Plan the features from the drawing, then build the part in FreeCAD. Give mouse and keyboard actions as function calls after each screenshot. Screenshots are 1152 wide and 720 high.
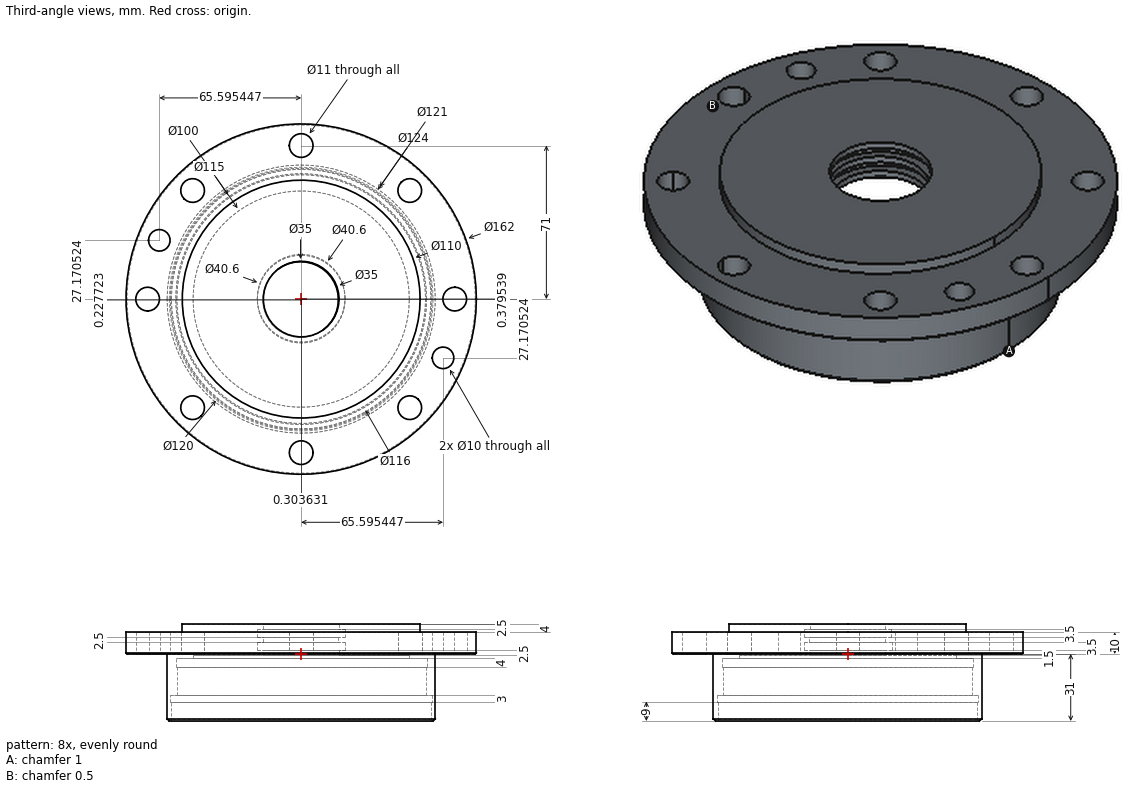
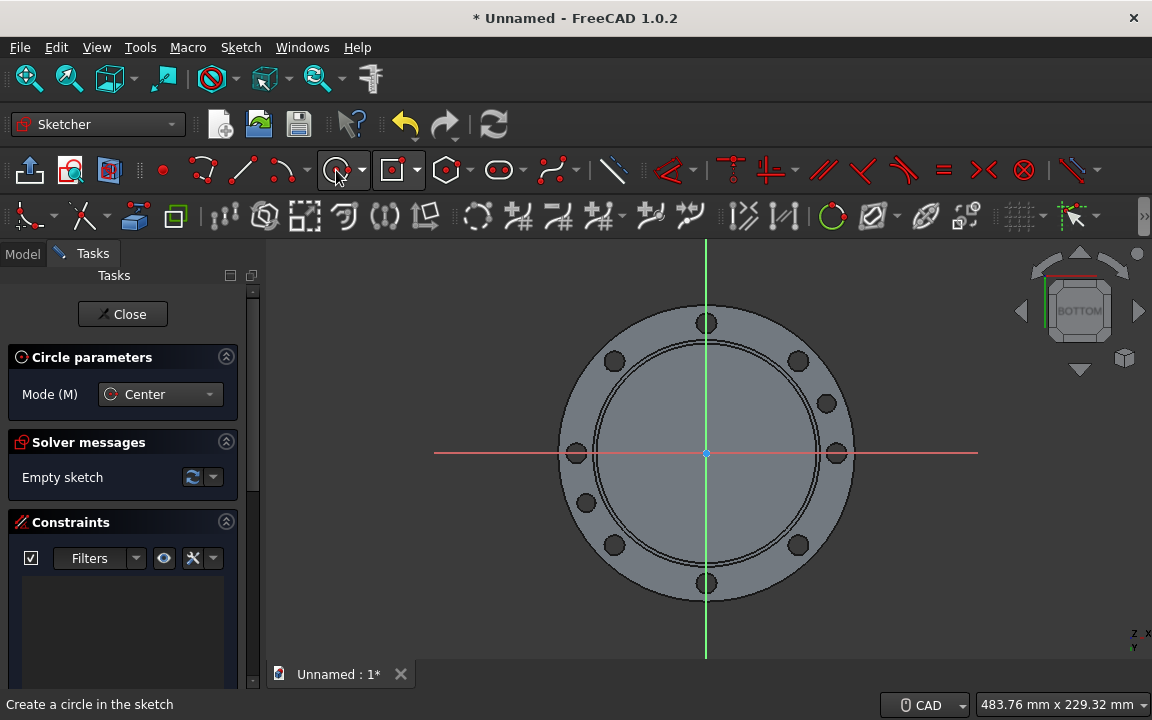
click(706, 453)
click(785, 375)
key(Escape)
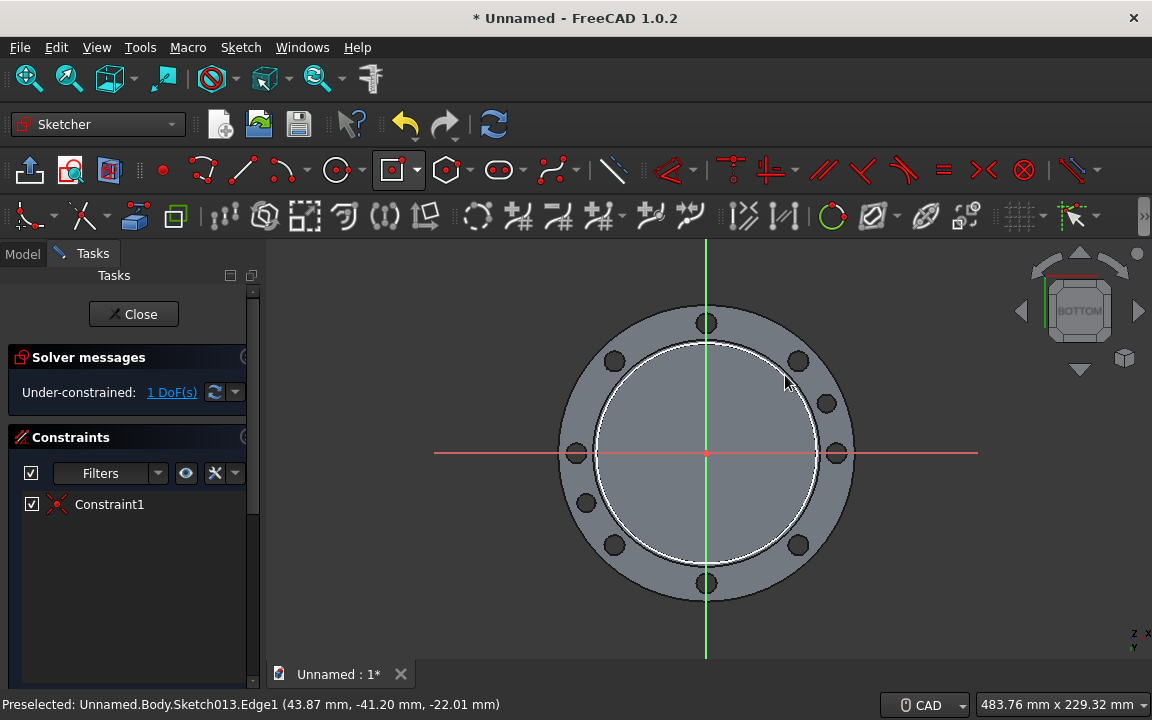
click(668, 170)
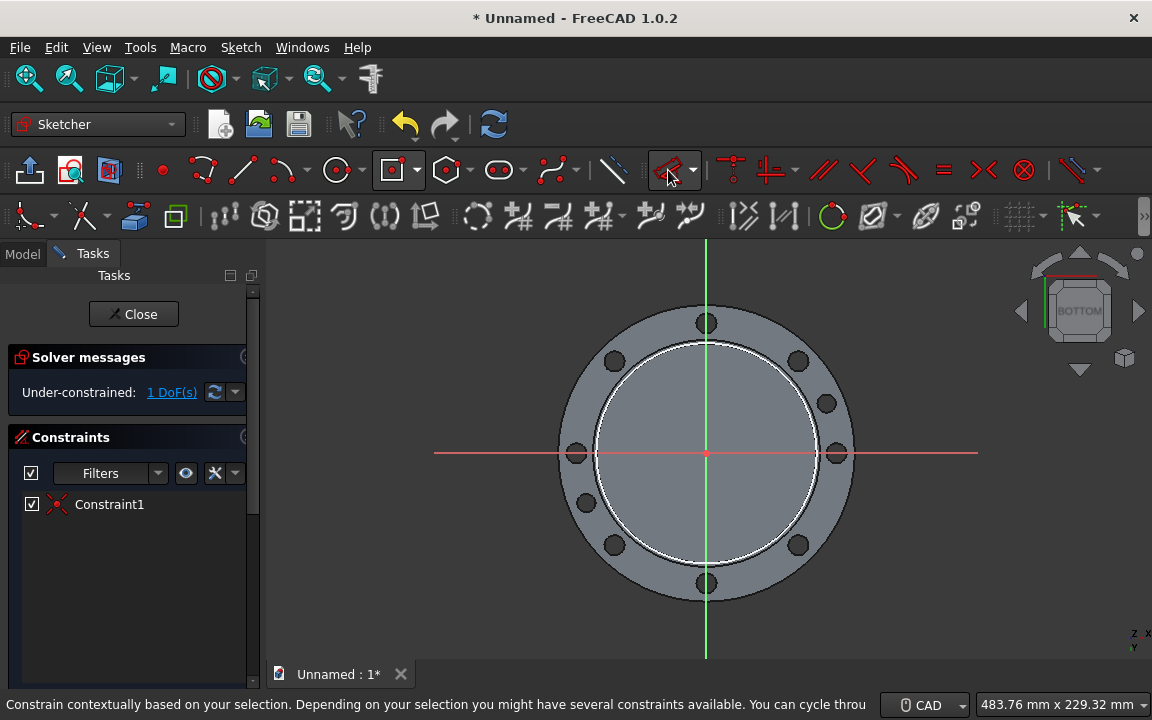
click(784, 375)
click(807, 352)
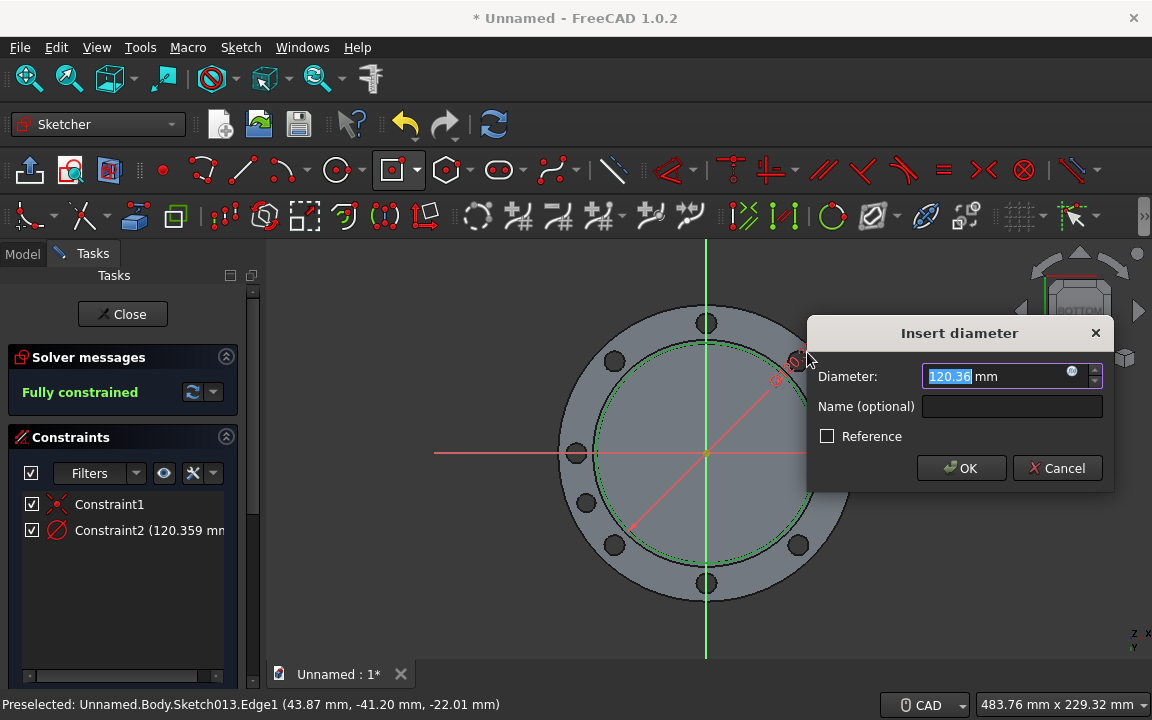
text(121)
key(Return)
key(Escape)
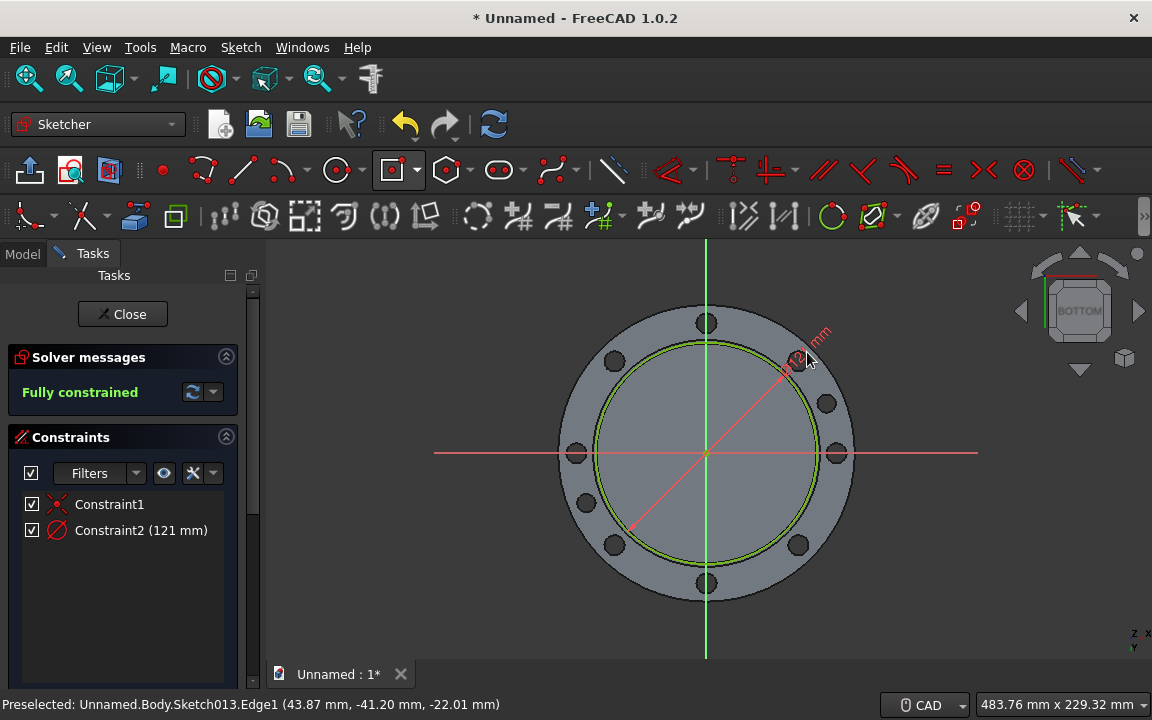
click(123, 314)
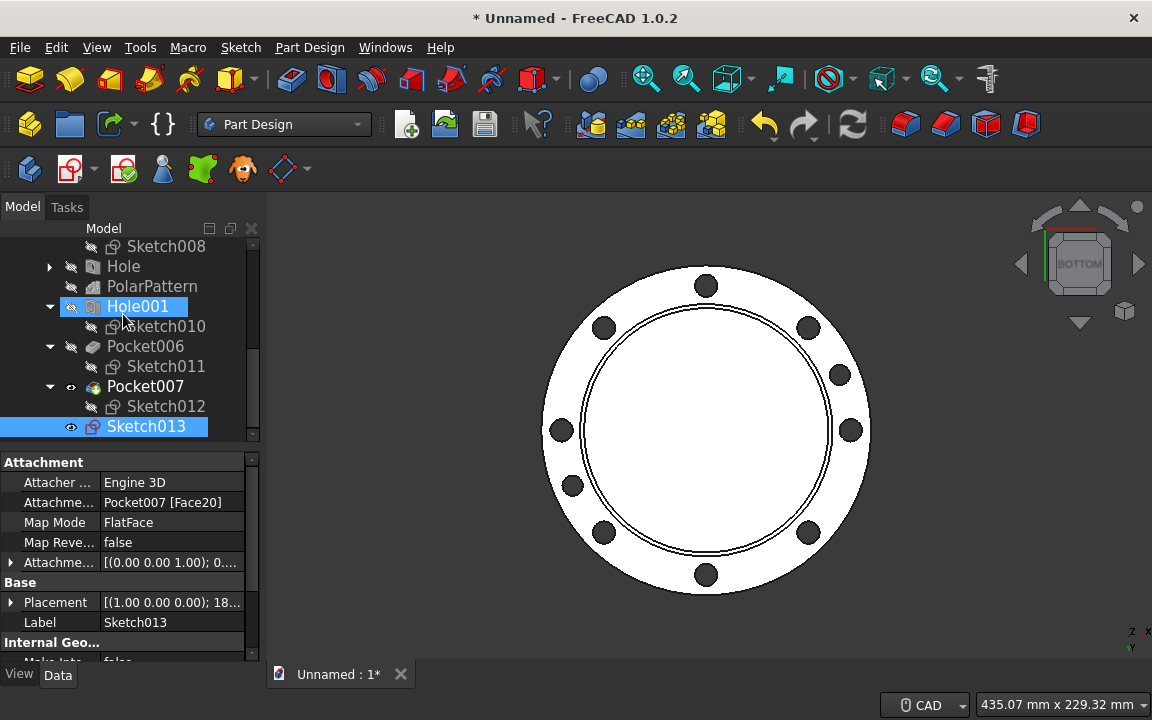
click(292, 80)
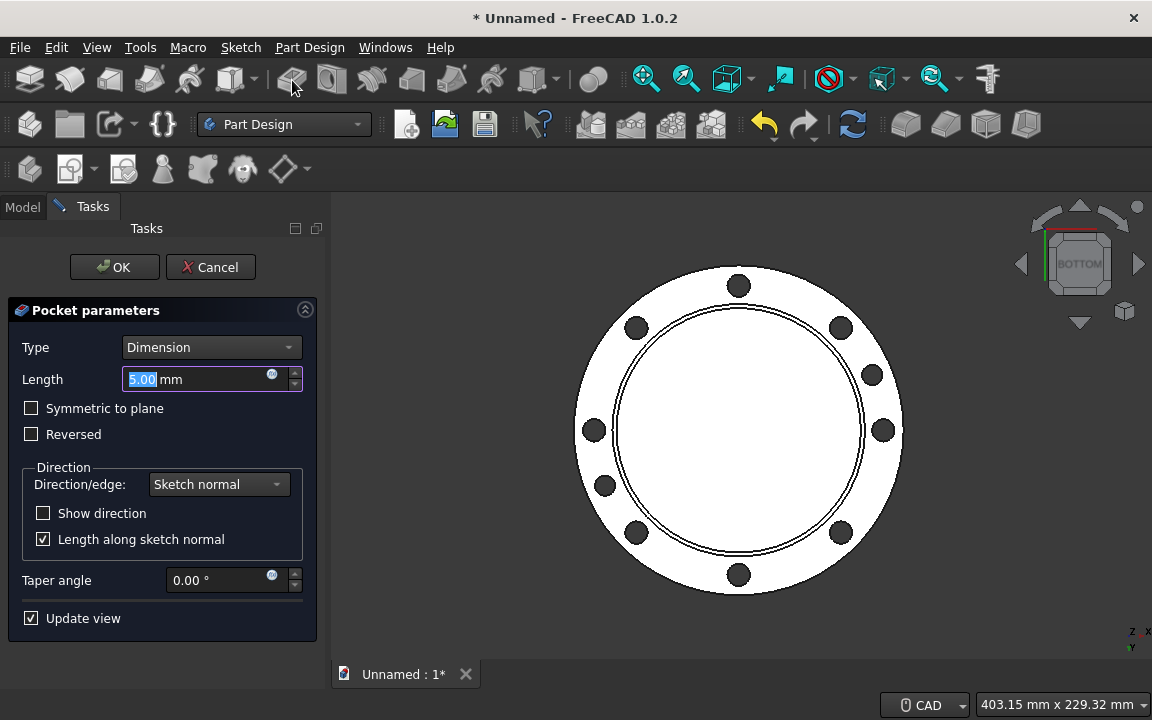
text(3)
key(Tab)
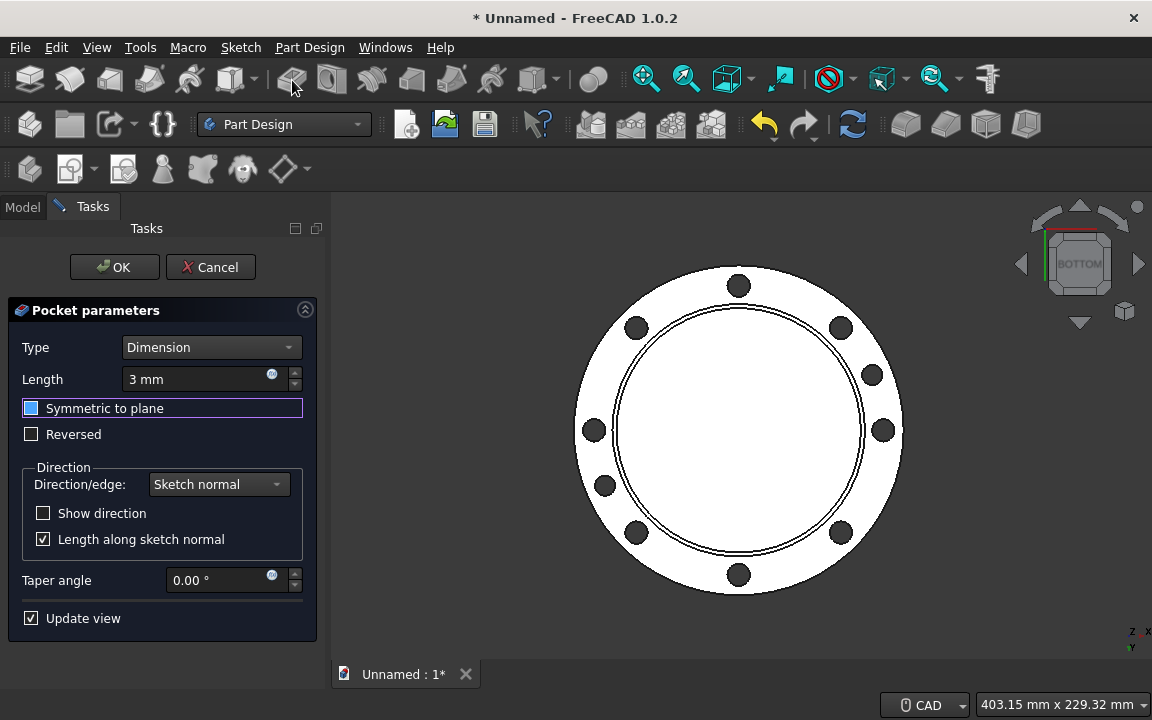
click(115, 267)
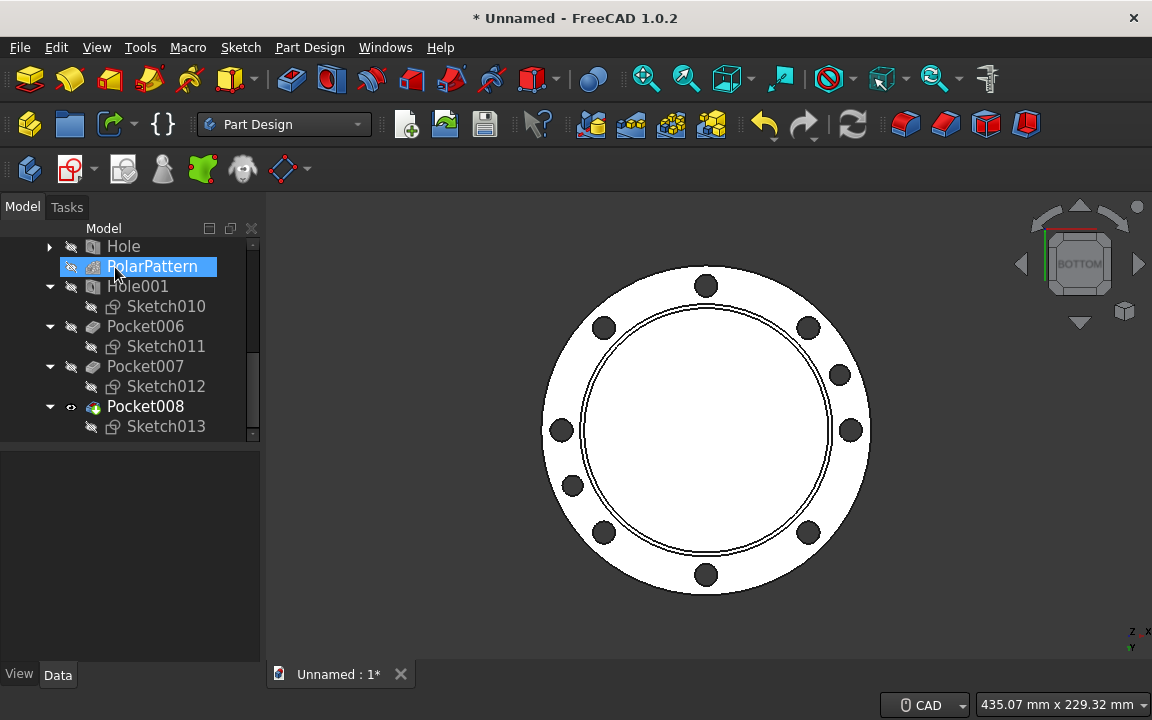
click(706, 429)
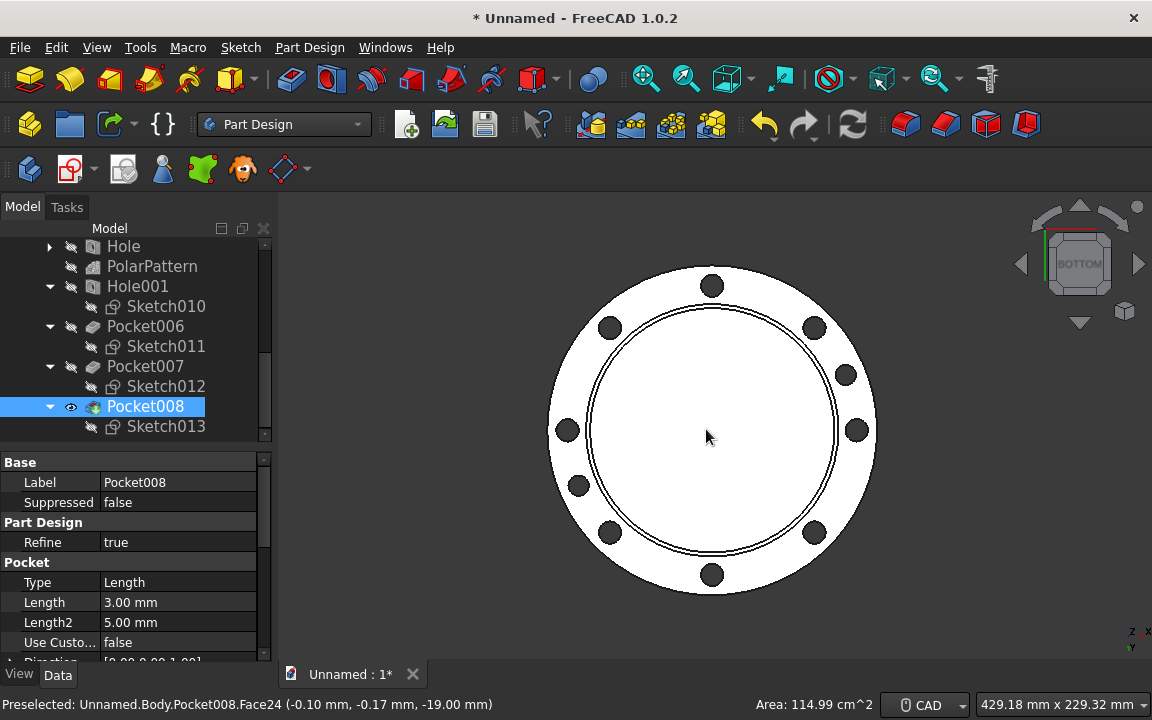
click(70, 170)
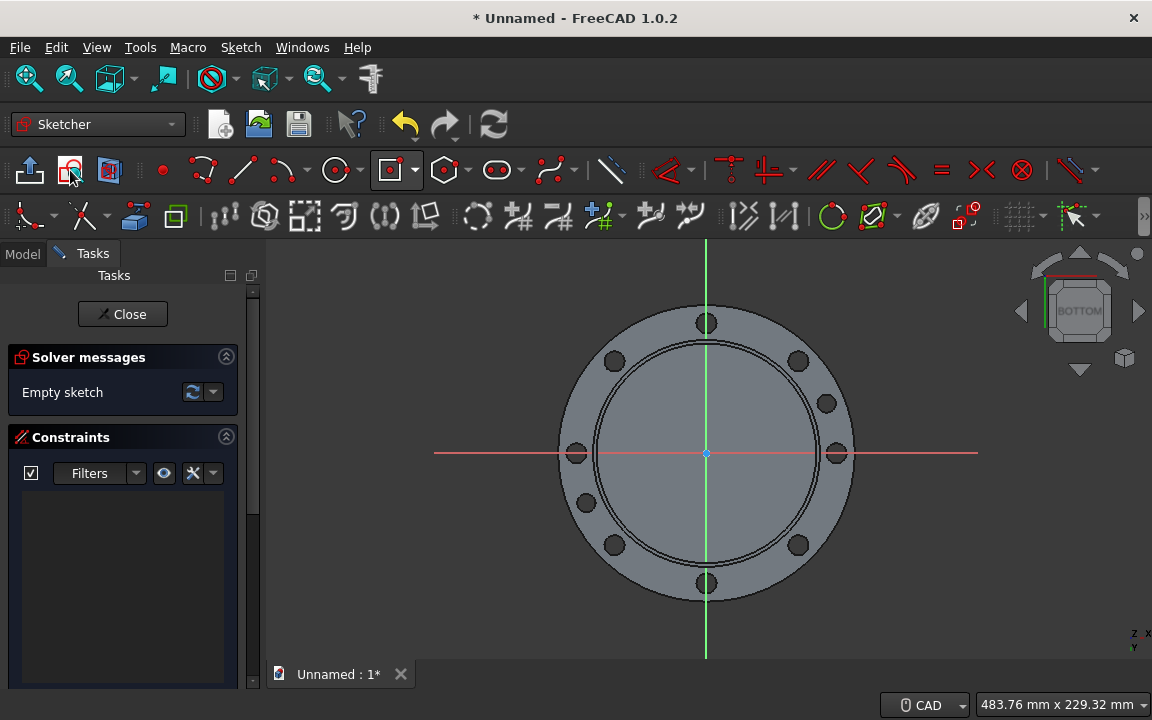
click(336, 170)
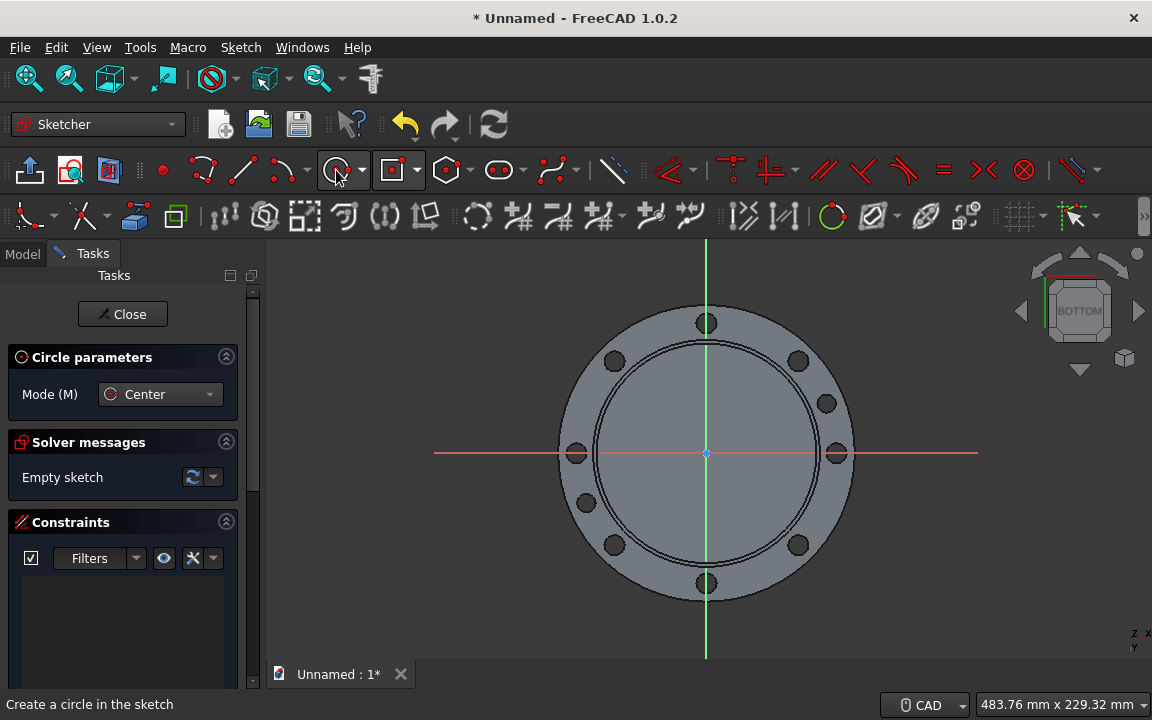
click(706, 453)
click(781, 379)
key(Escape)